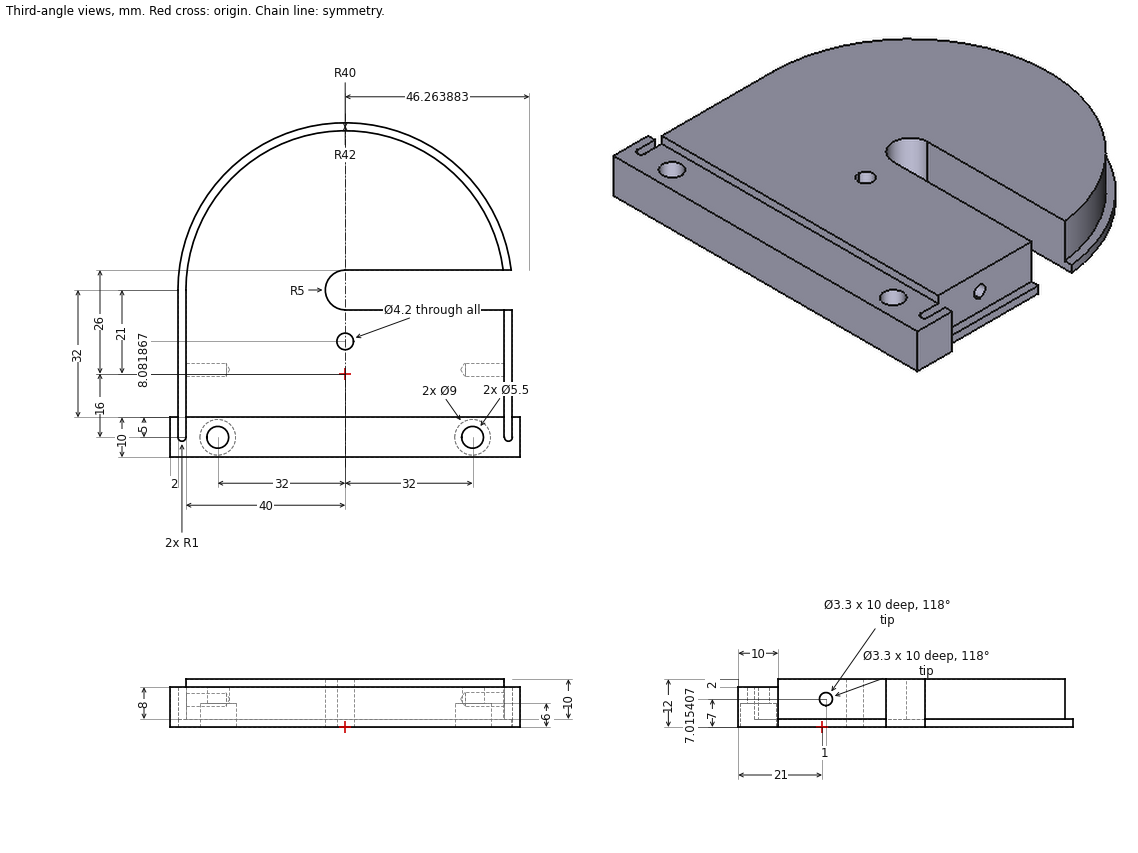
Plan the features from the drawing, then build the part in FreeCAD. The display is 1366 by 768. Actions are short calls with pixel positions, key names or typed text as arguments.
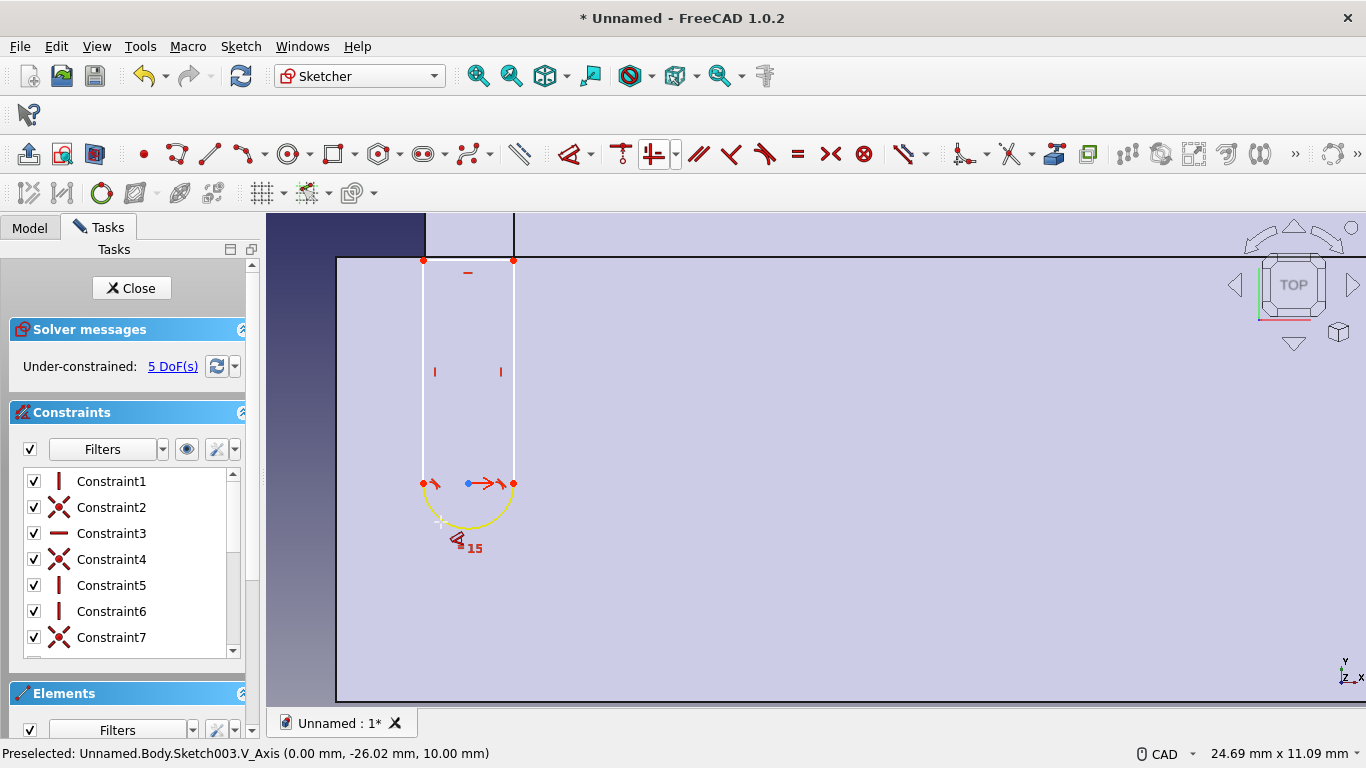
click(442, 520)
click(423, 546)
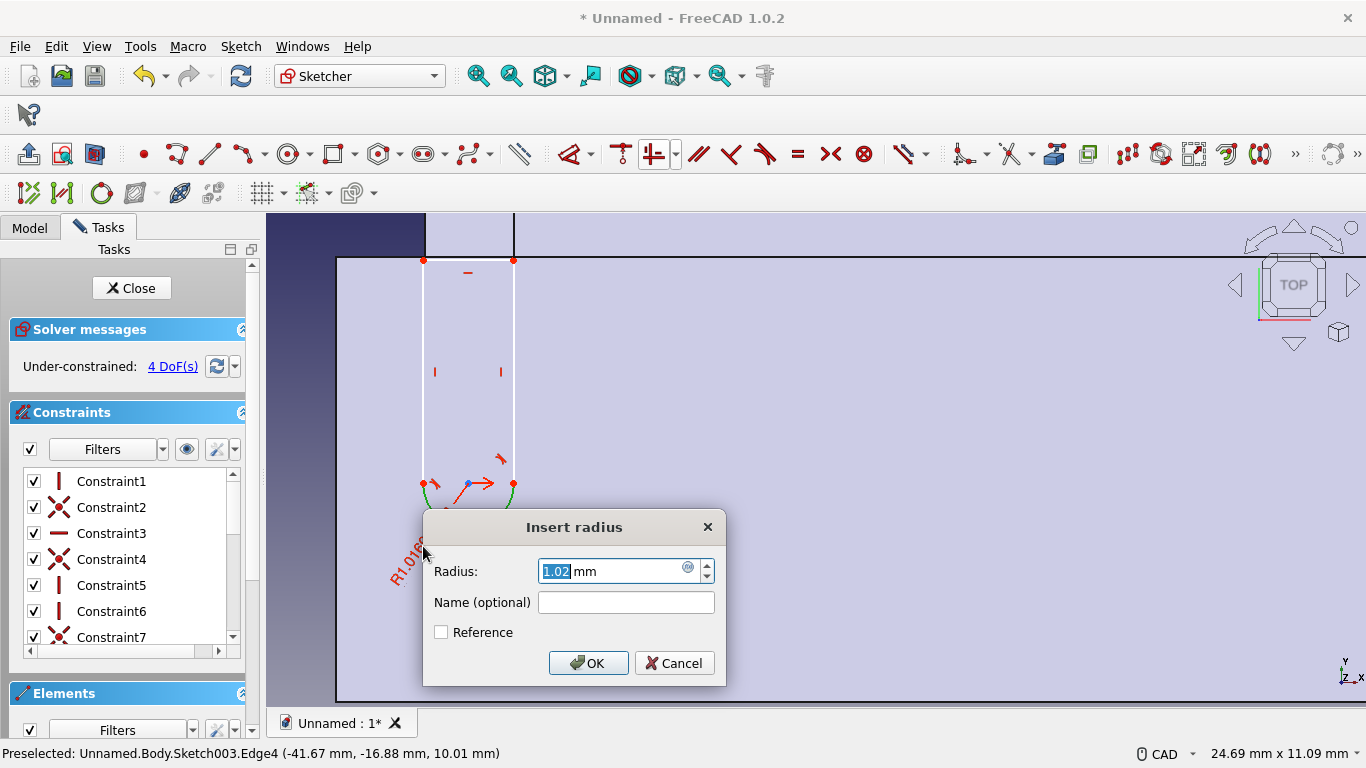
text(1)
key(Return)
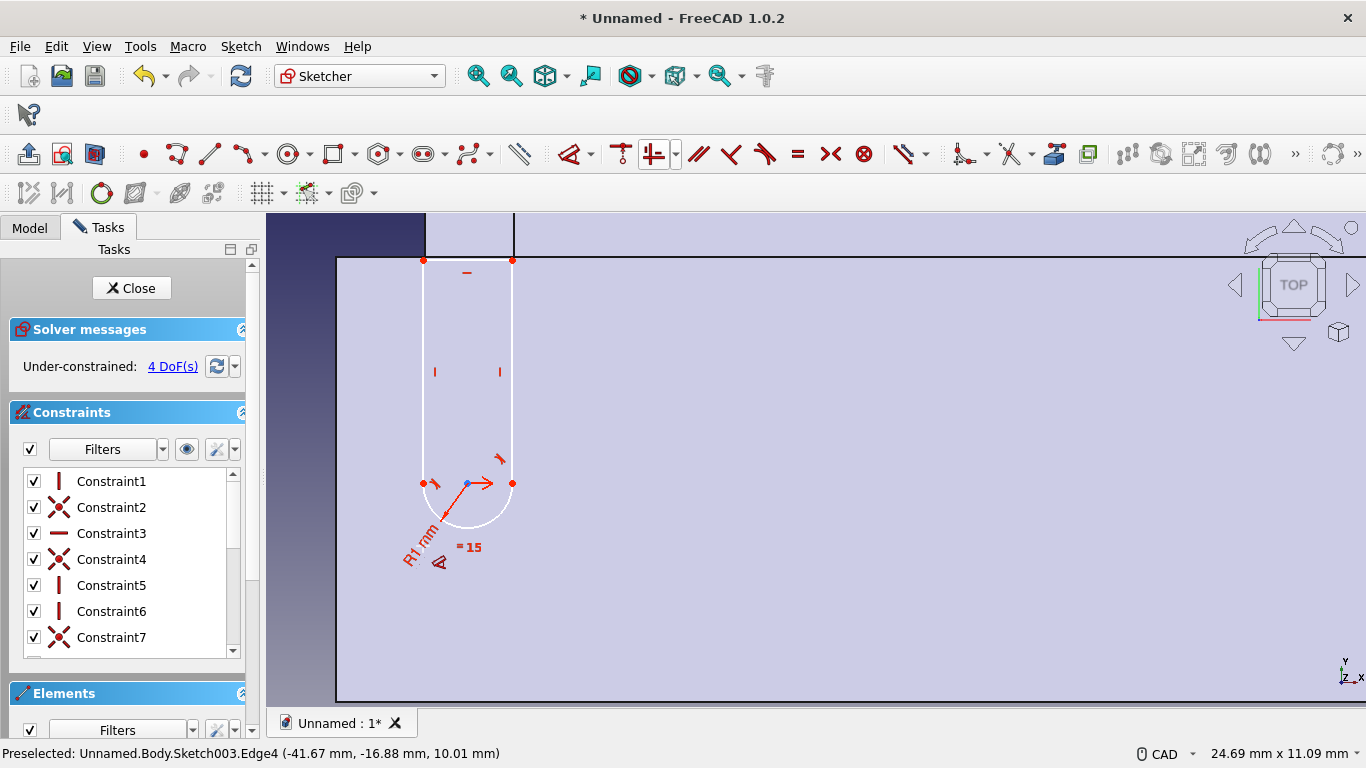
scroll(441, 522, down, 9)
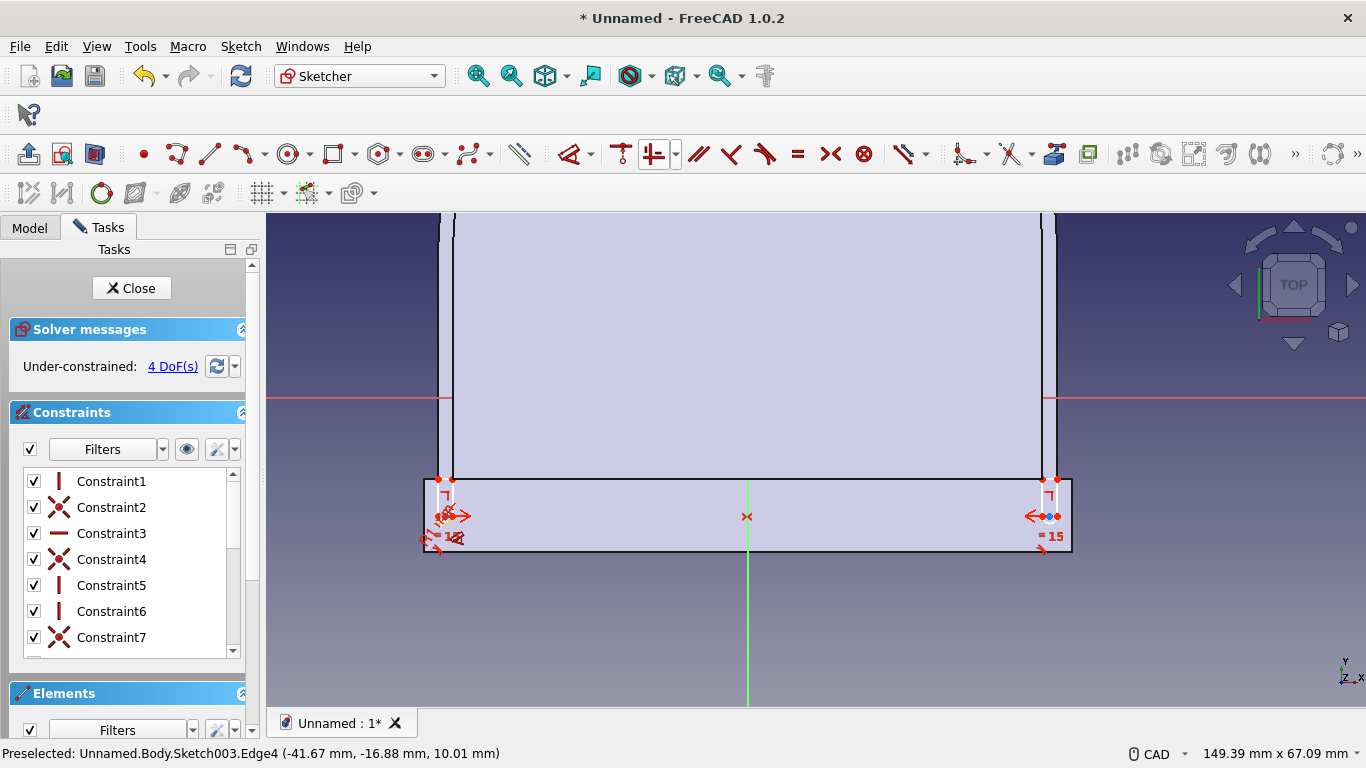
scroll(453, 505, up, 2)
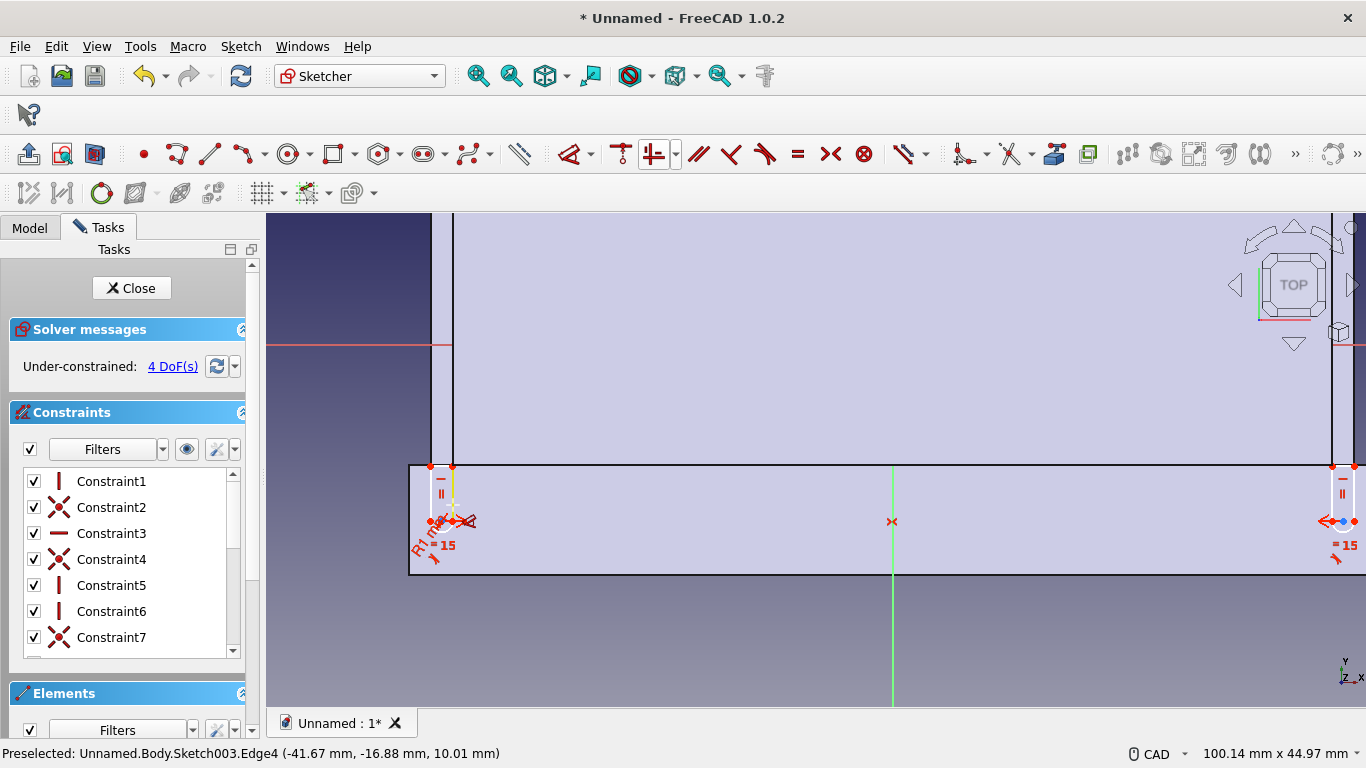
click(453, 505)
click(487, 494)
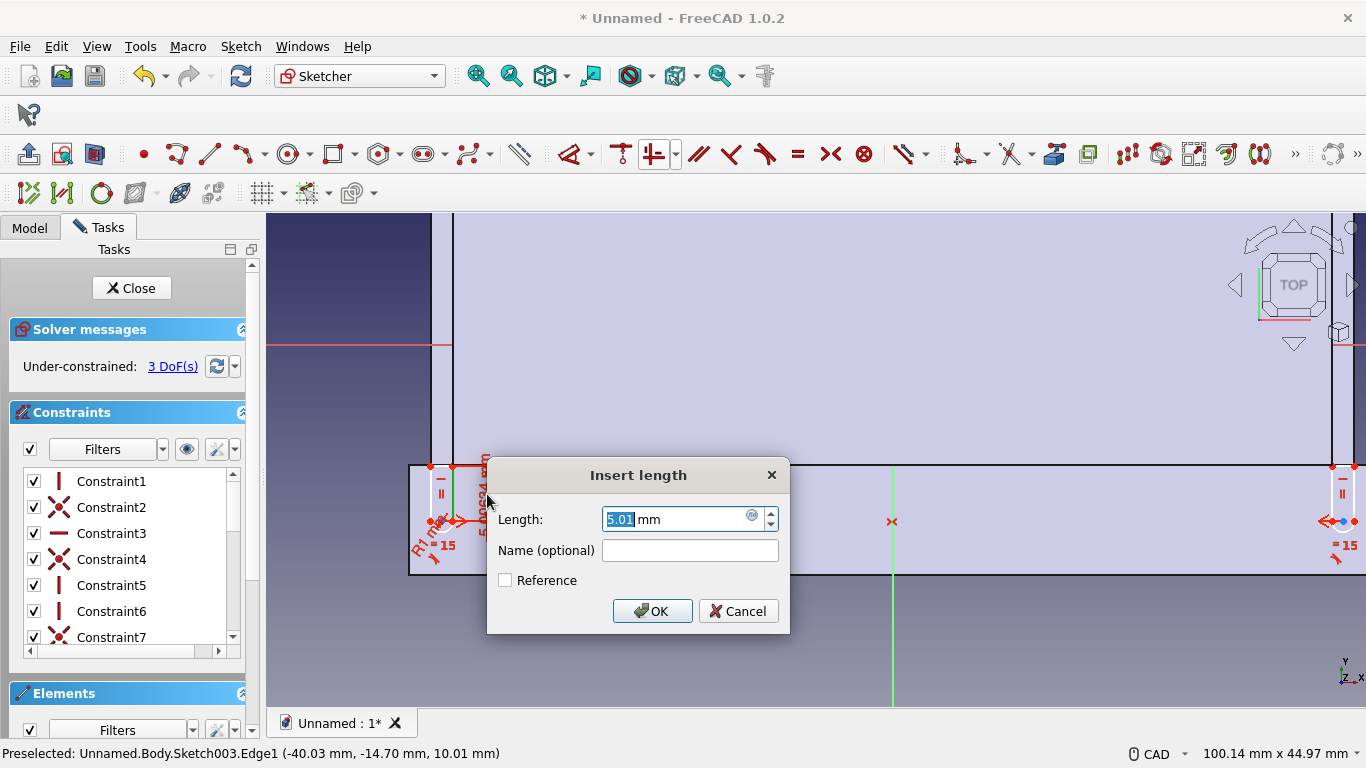
text(5)
key(Return)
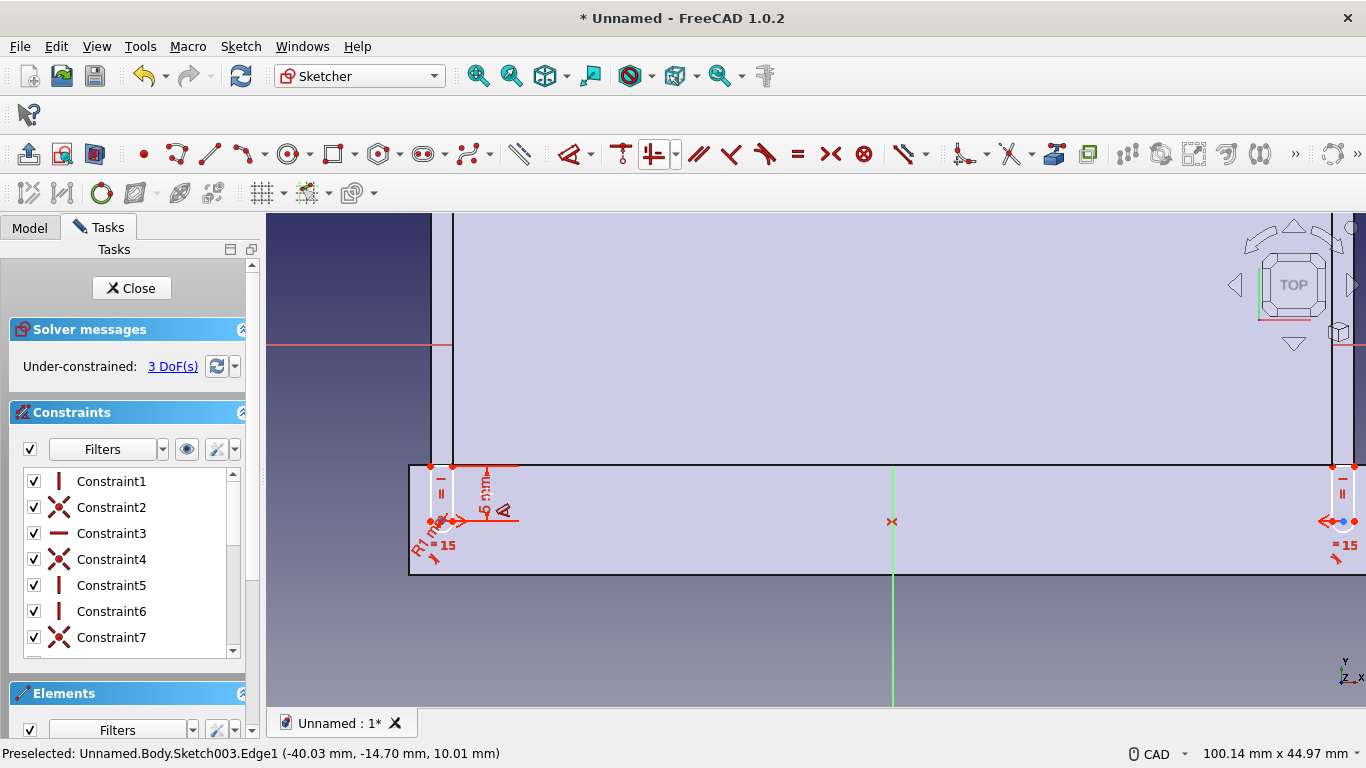
scroll(453, 505, down, 2)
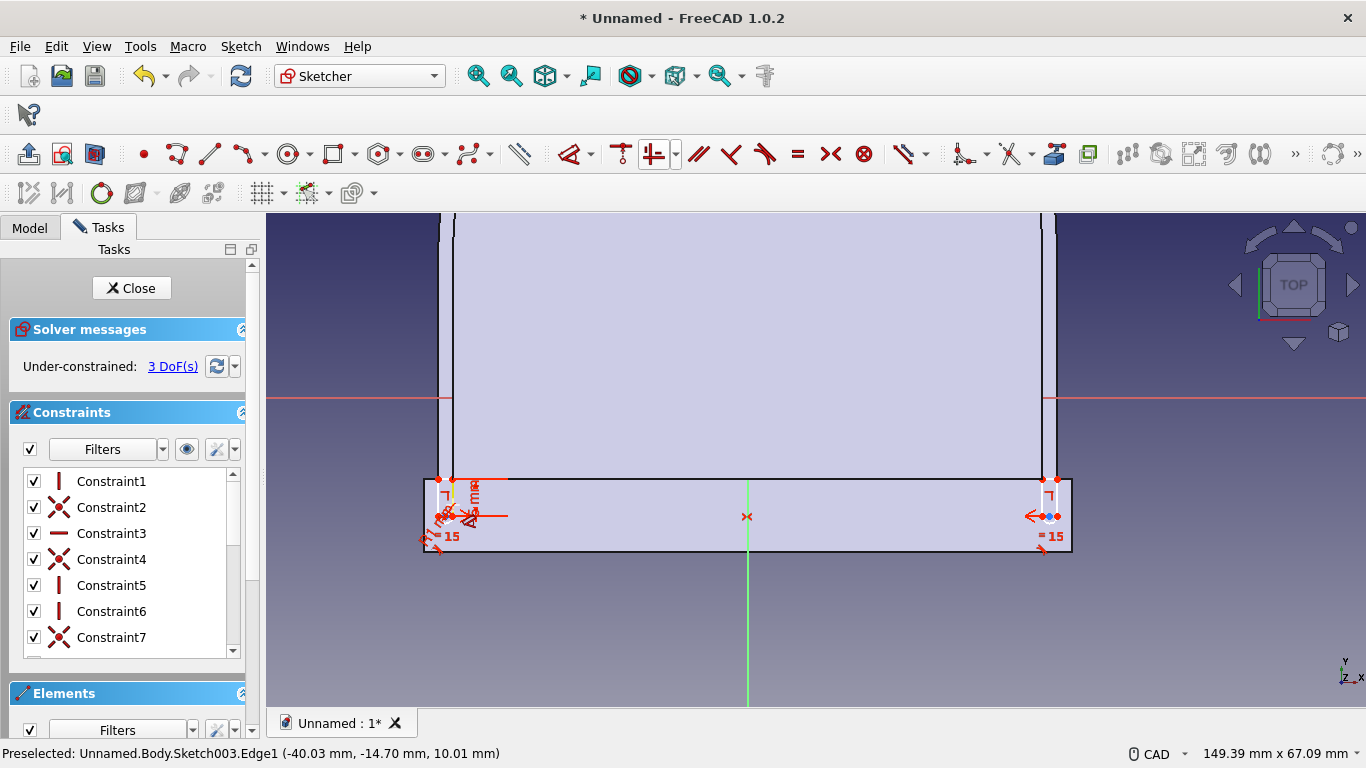
scroll(1057, 505, up, 2)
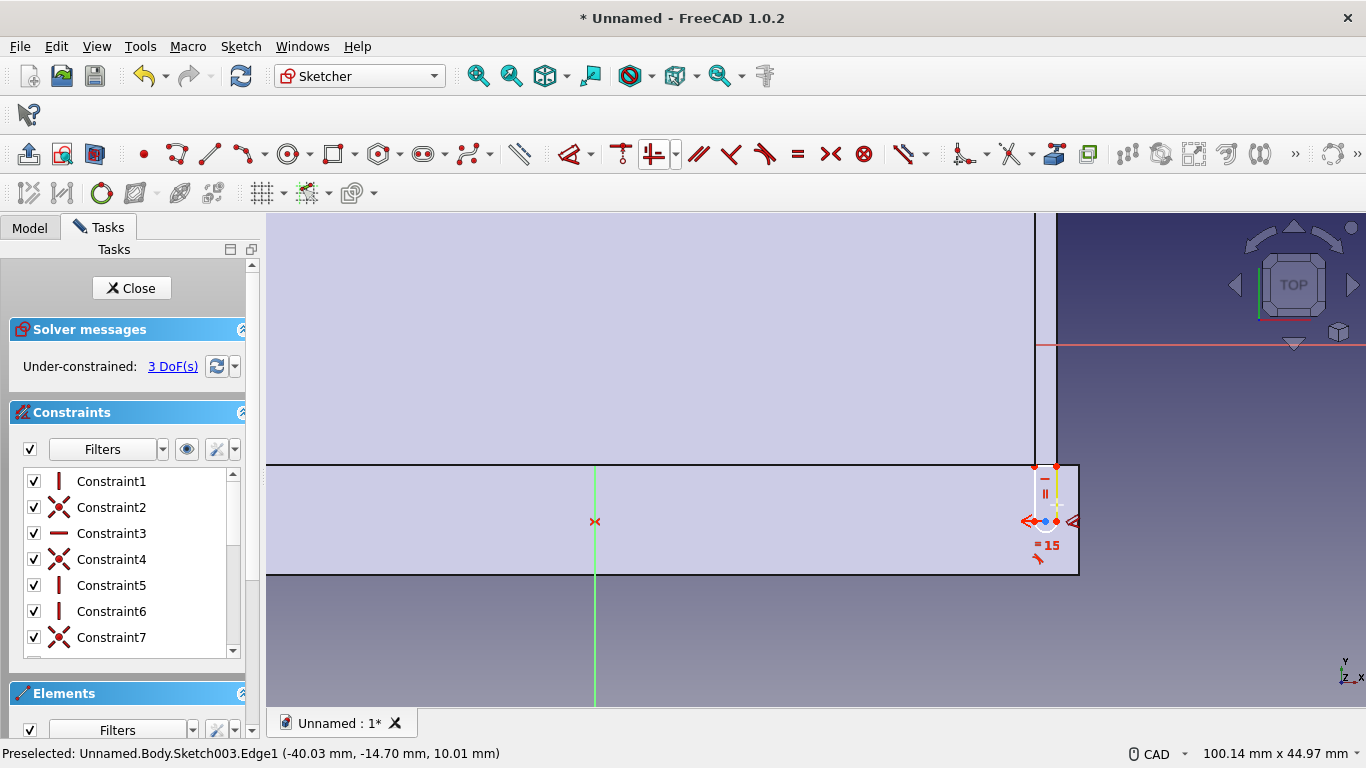
click(1057, 505)
click(1091, 494)